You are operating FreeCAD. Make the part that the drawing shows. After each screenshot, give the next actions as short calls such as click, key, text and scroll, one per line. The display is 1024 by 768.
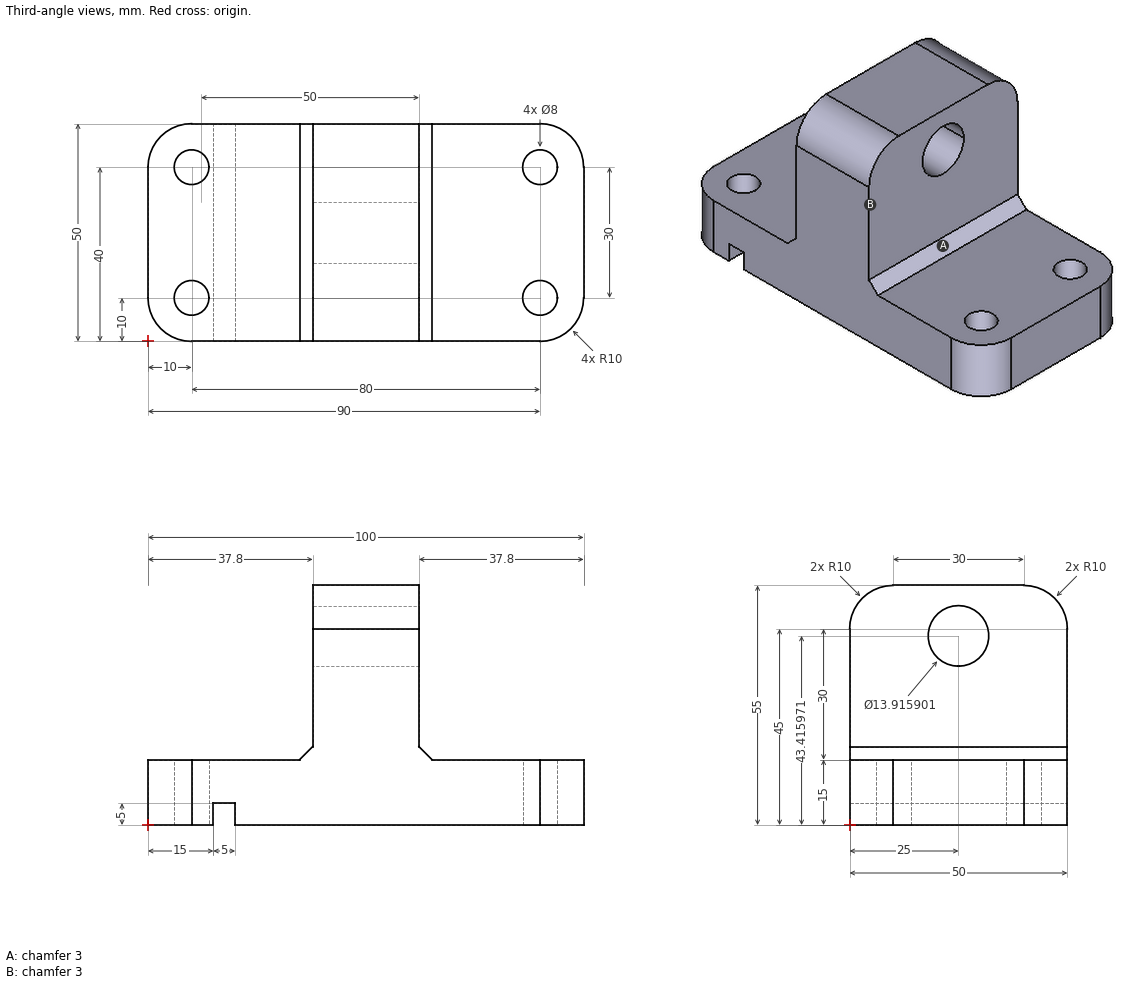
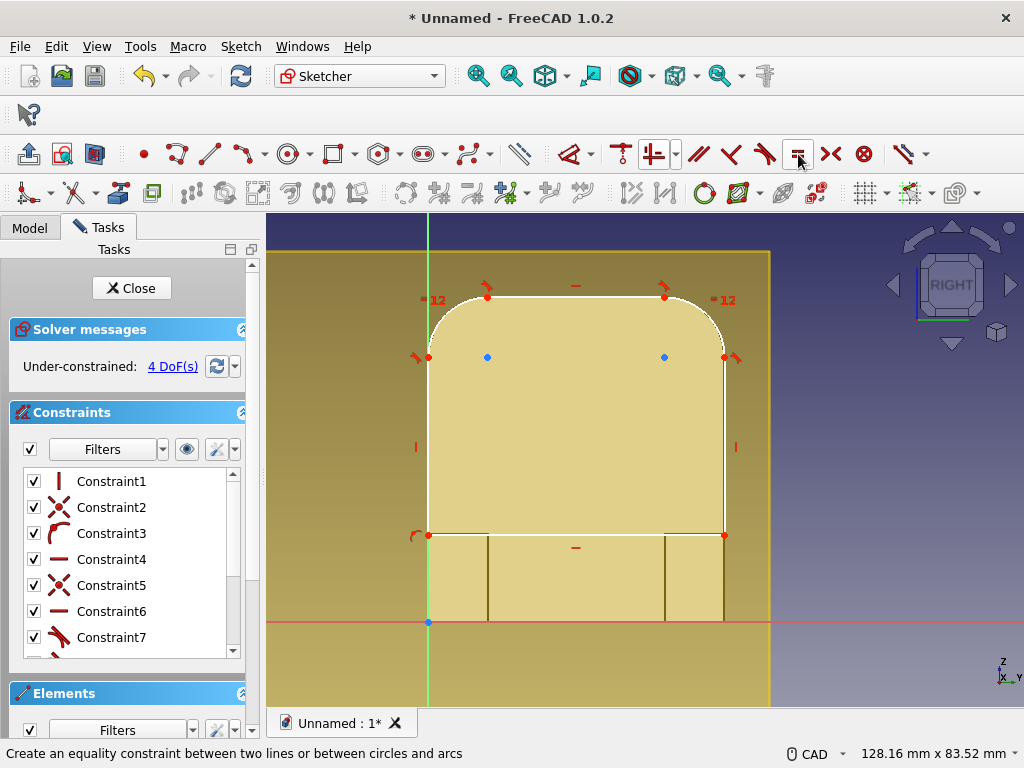
click(568, 154)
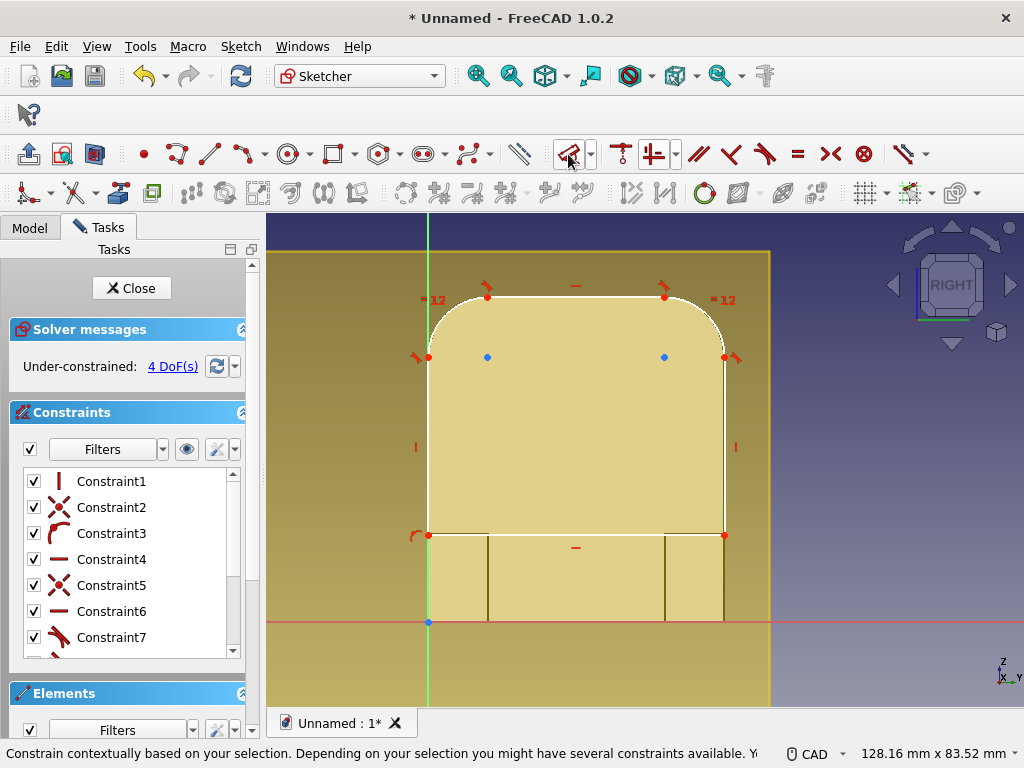
click(461, 304)
click(446, 275)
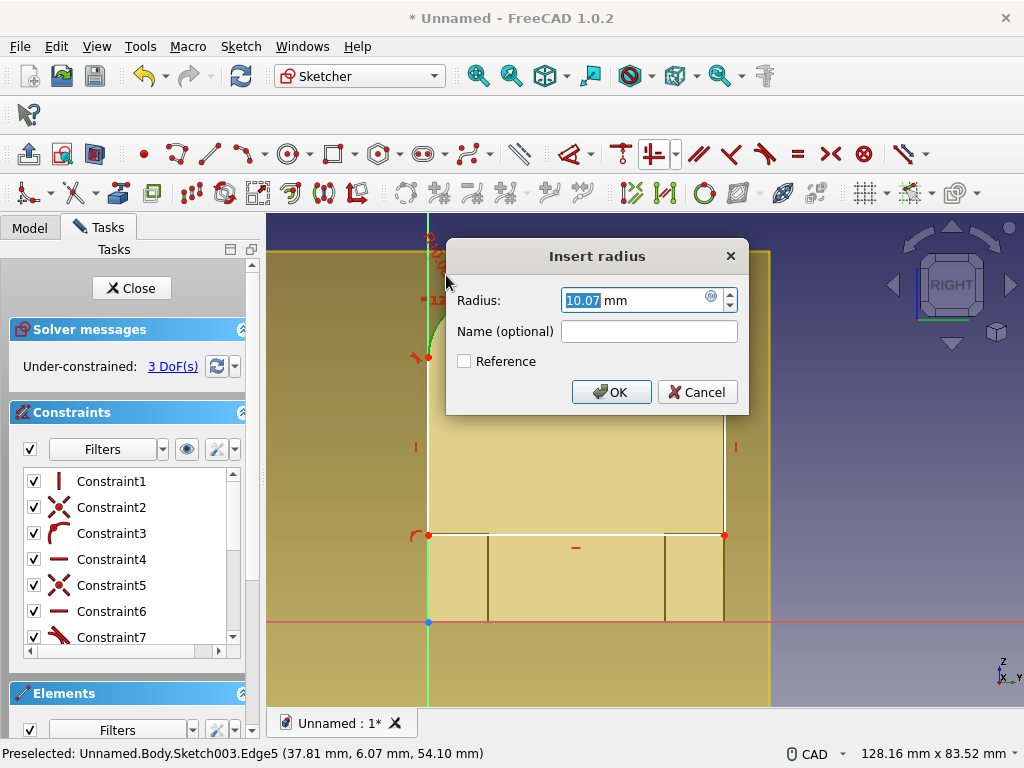
text(10)
key(Return)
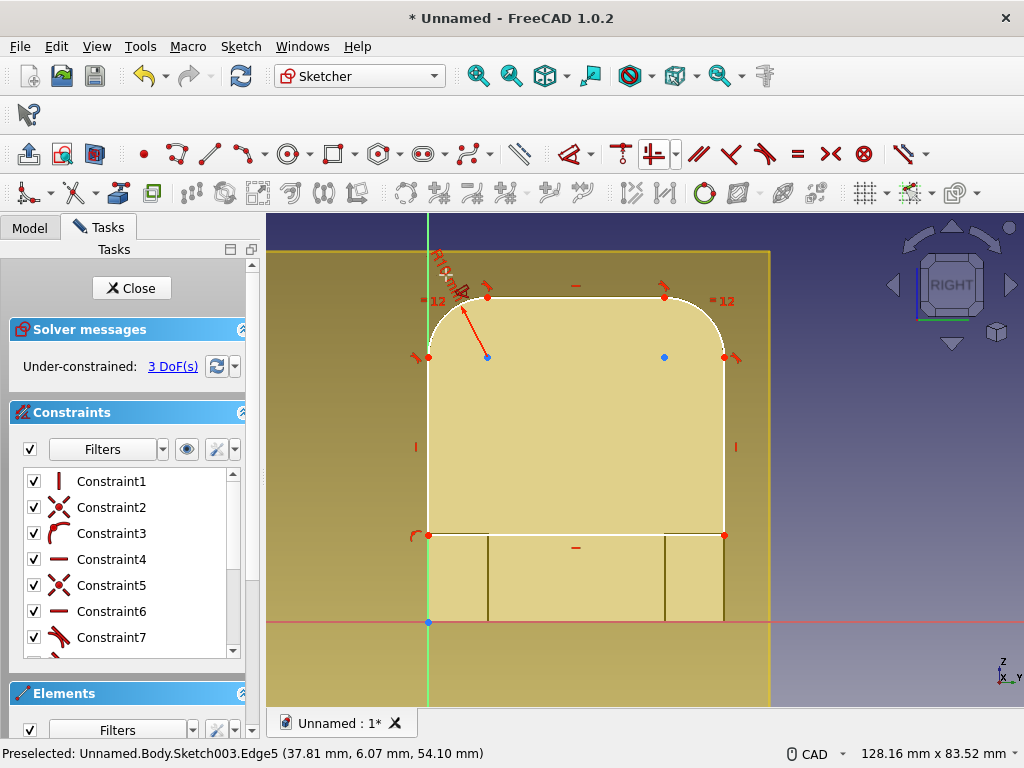
click(724, 410)
click(758, 446)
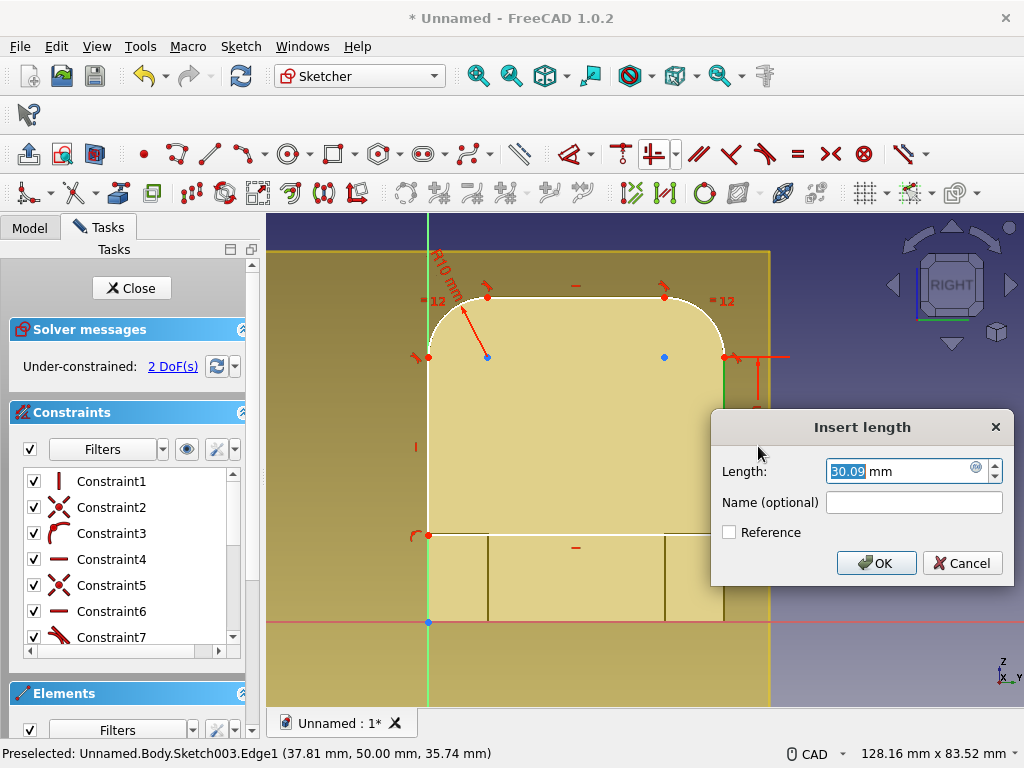
text(30)
key(Return)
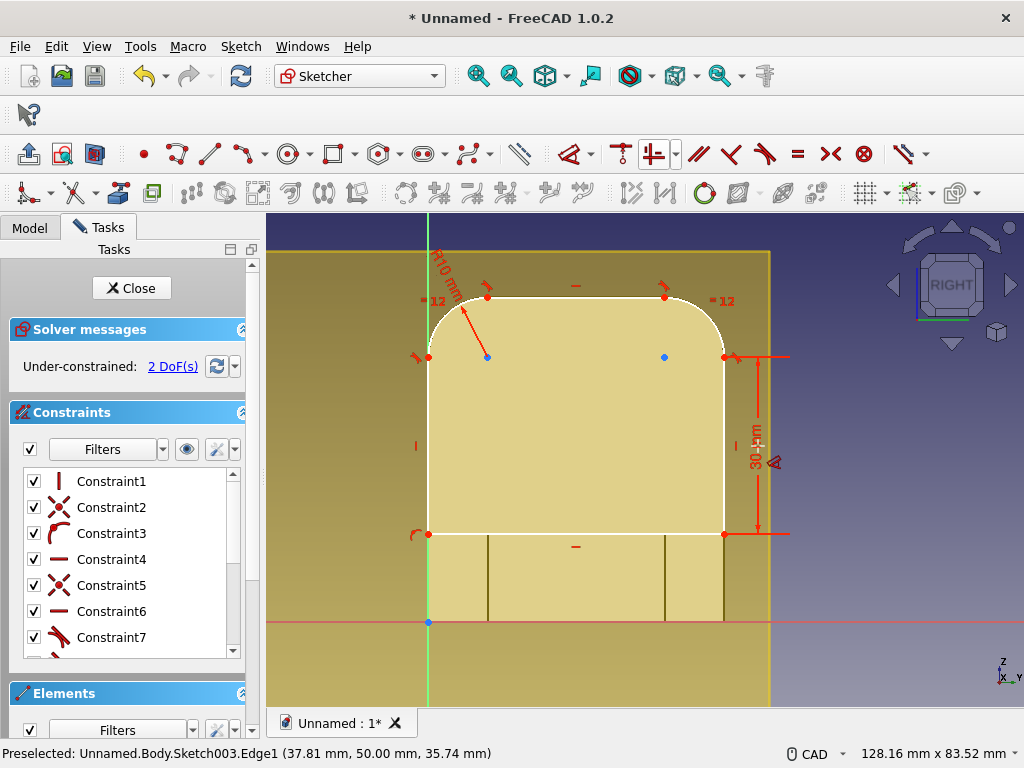
click(635, 534)
click(576, 568)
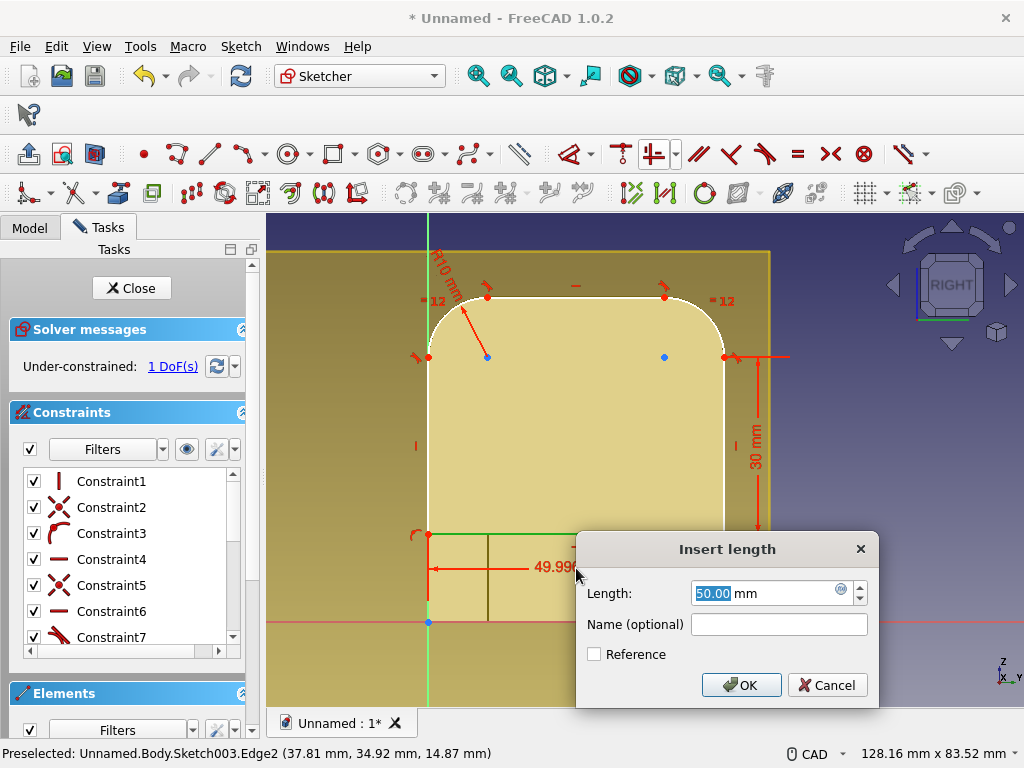
text(50)
key(Return)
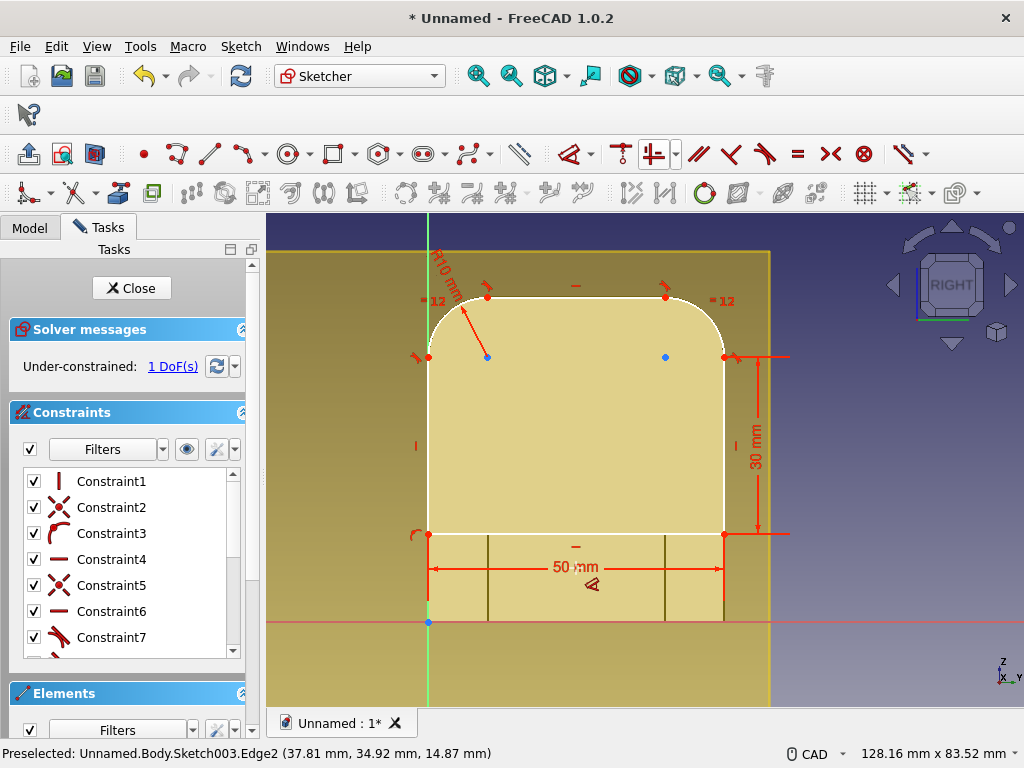
click(724, 357)
click(758, 490)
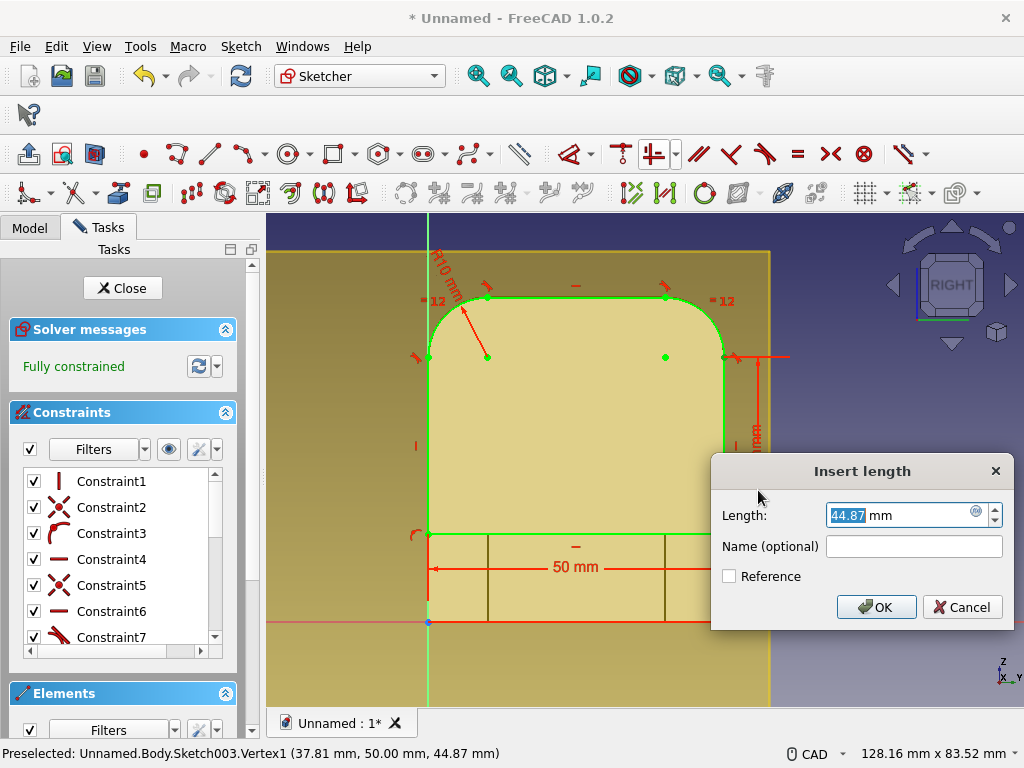
text(45)
key(Return)
key(Escape)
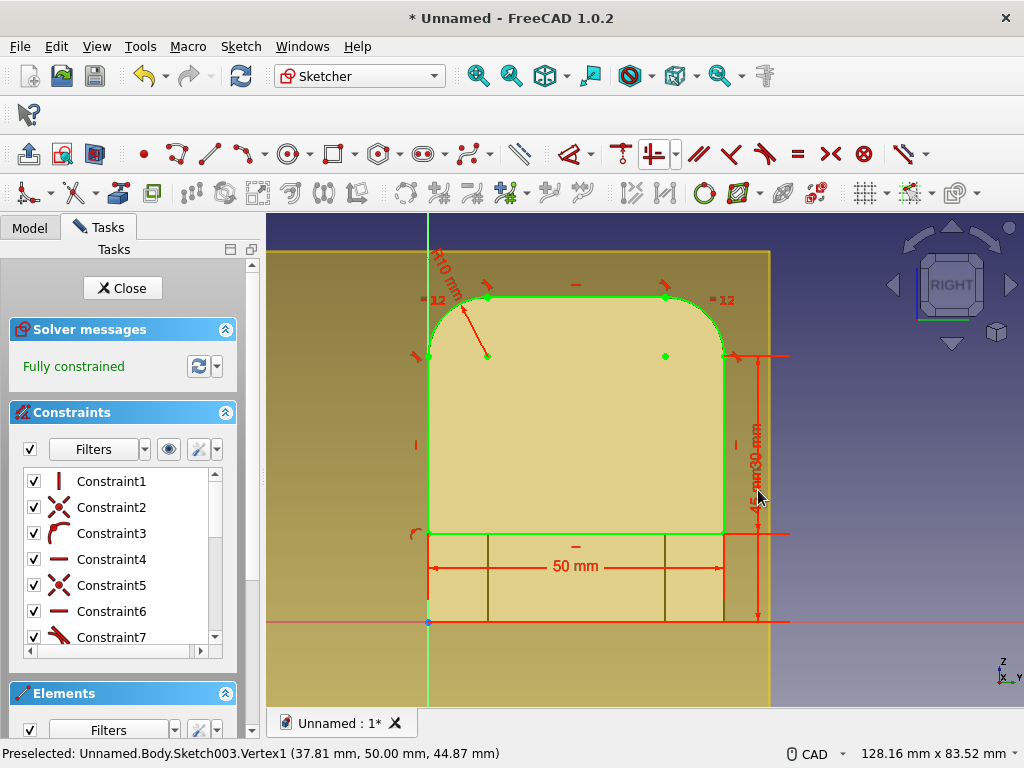
click(123, 288)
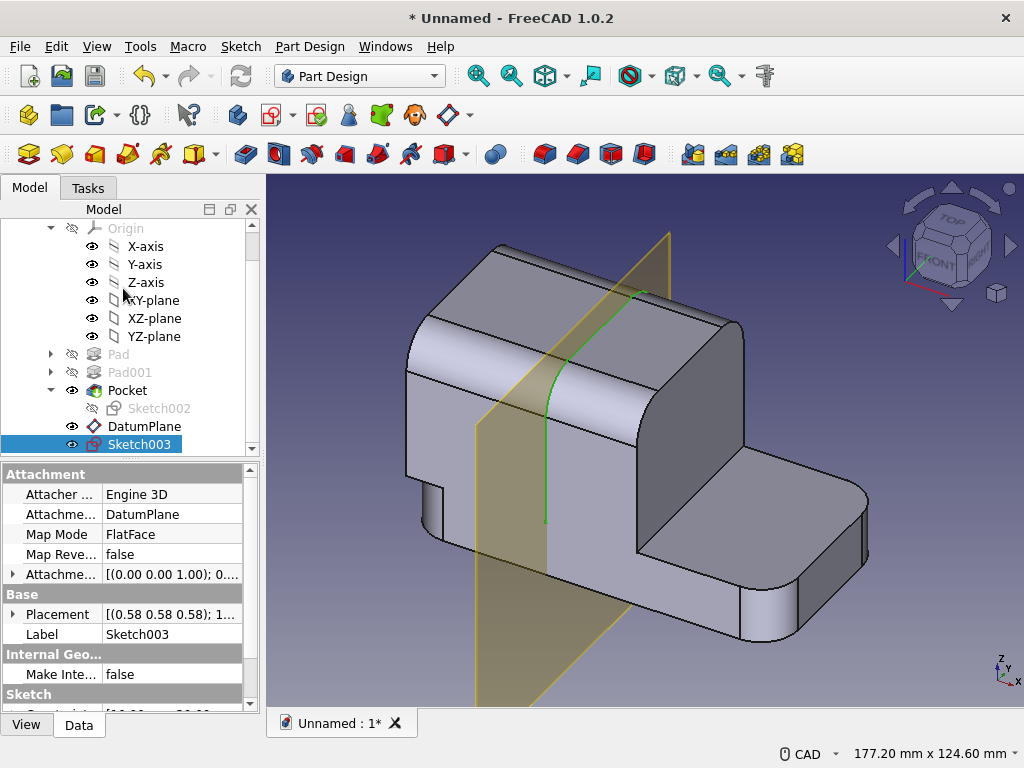
click(246, 154)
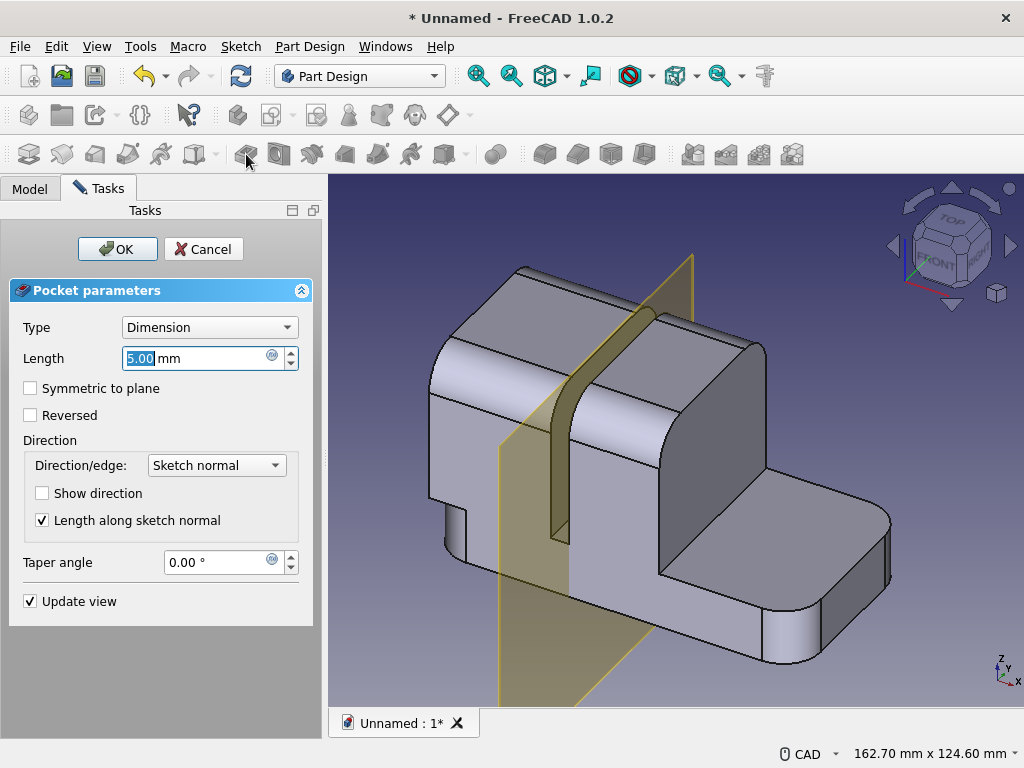
text(37.8)
key(Tab)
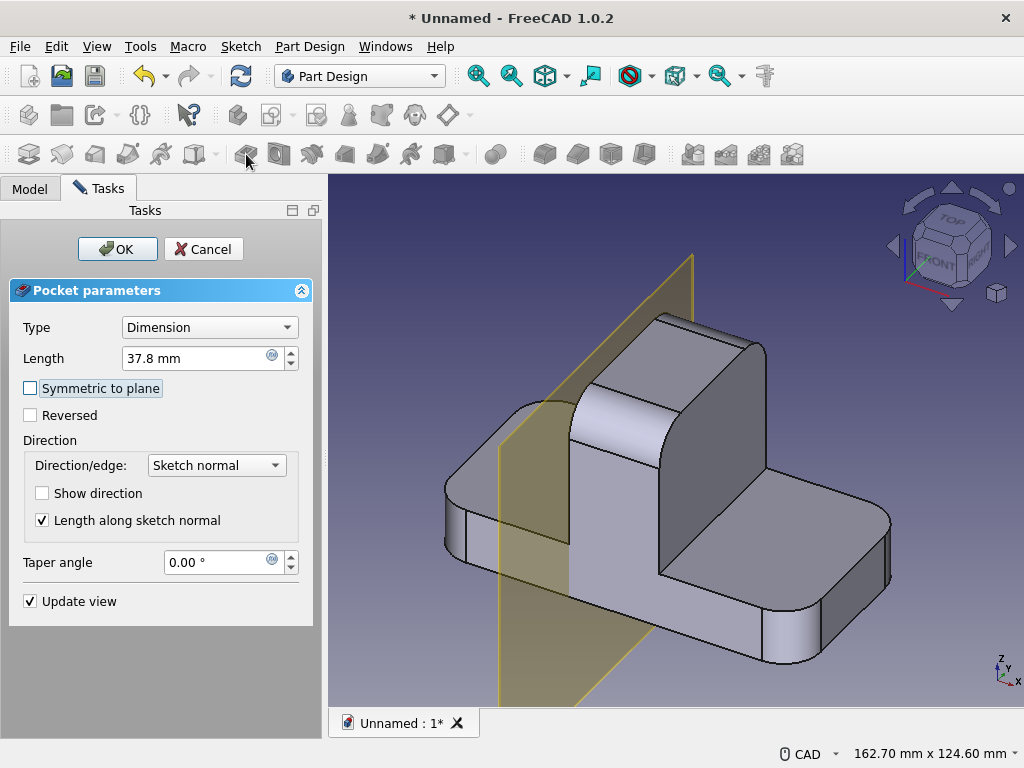
click(118, 249)